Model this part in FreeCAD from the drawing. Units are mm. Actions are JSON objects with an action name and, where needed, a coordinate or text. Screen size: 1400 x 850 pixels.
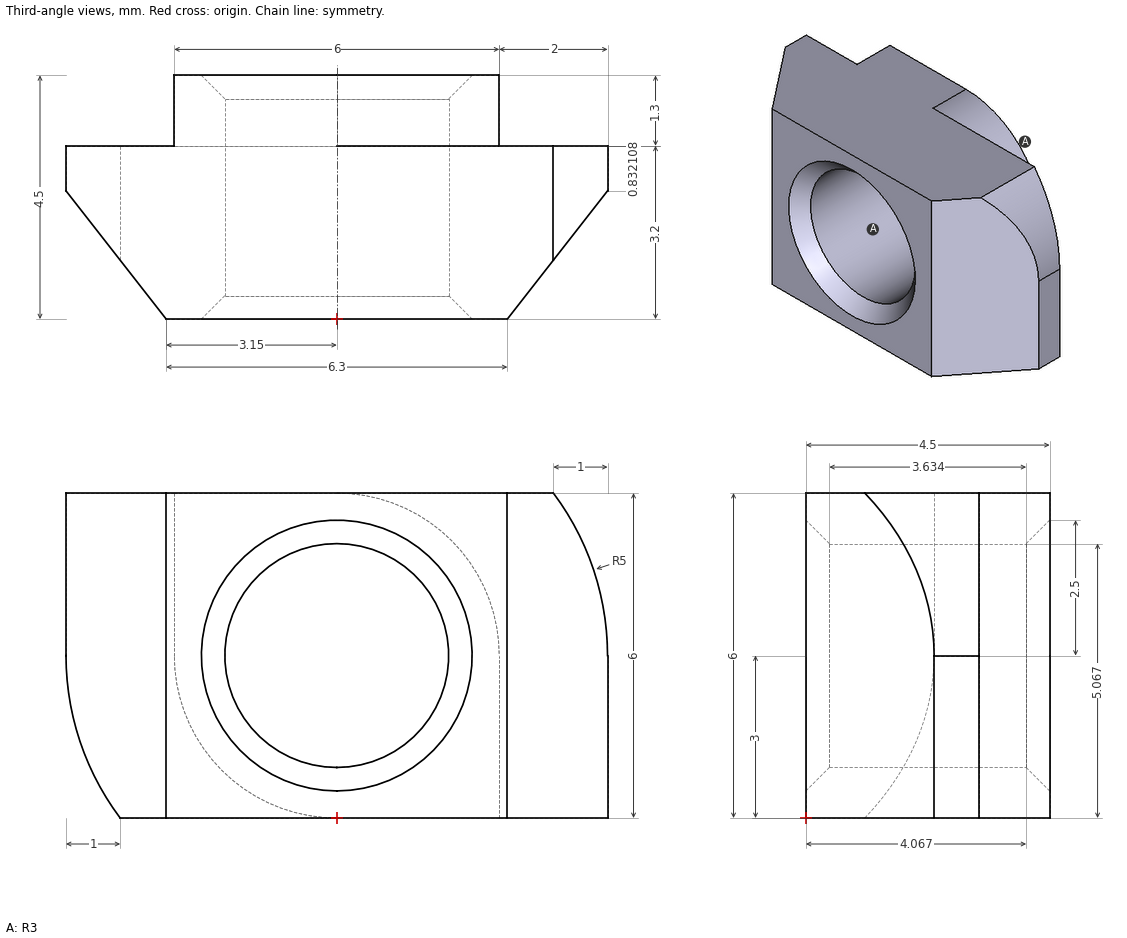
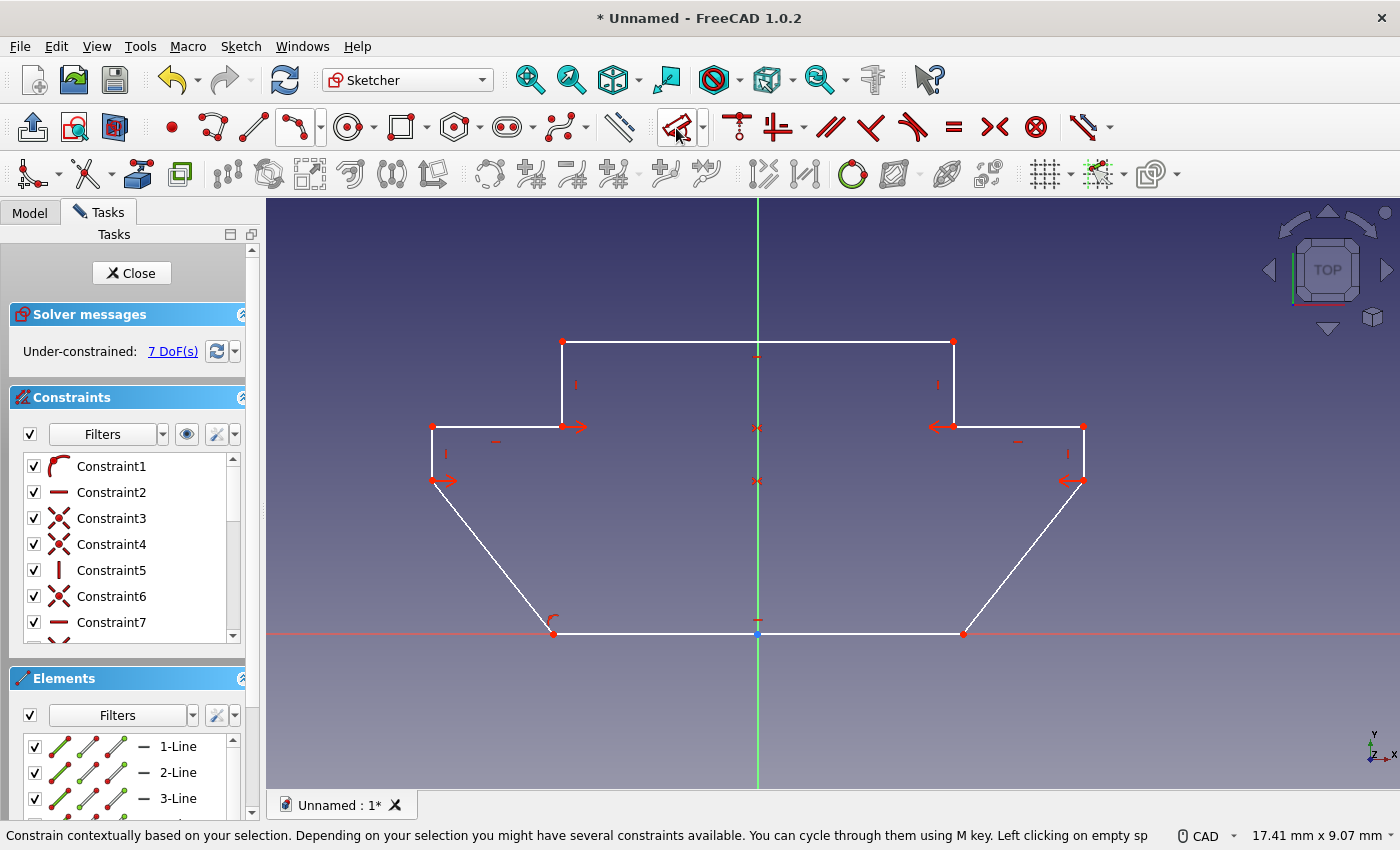
{"action": "left_click", "coordinate": [1045, 427]}
{"action": "left_click", "coordinate": [1019, 393]}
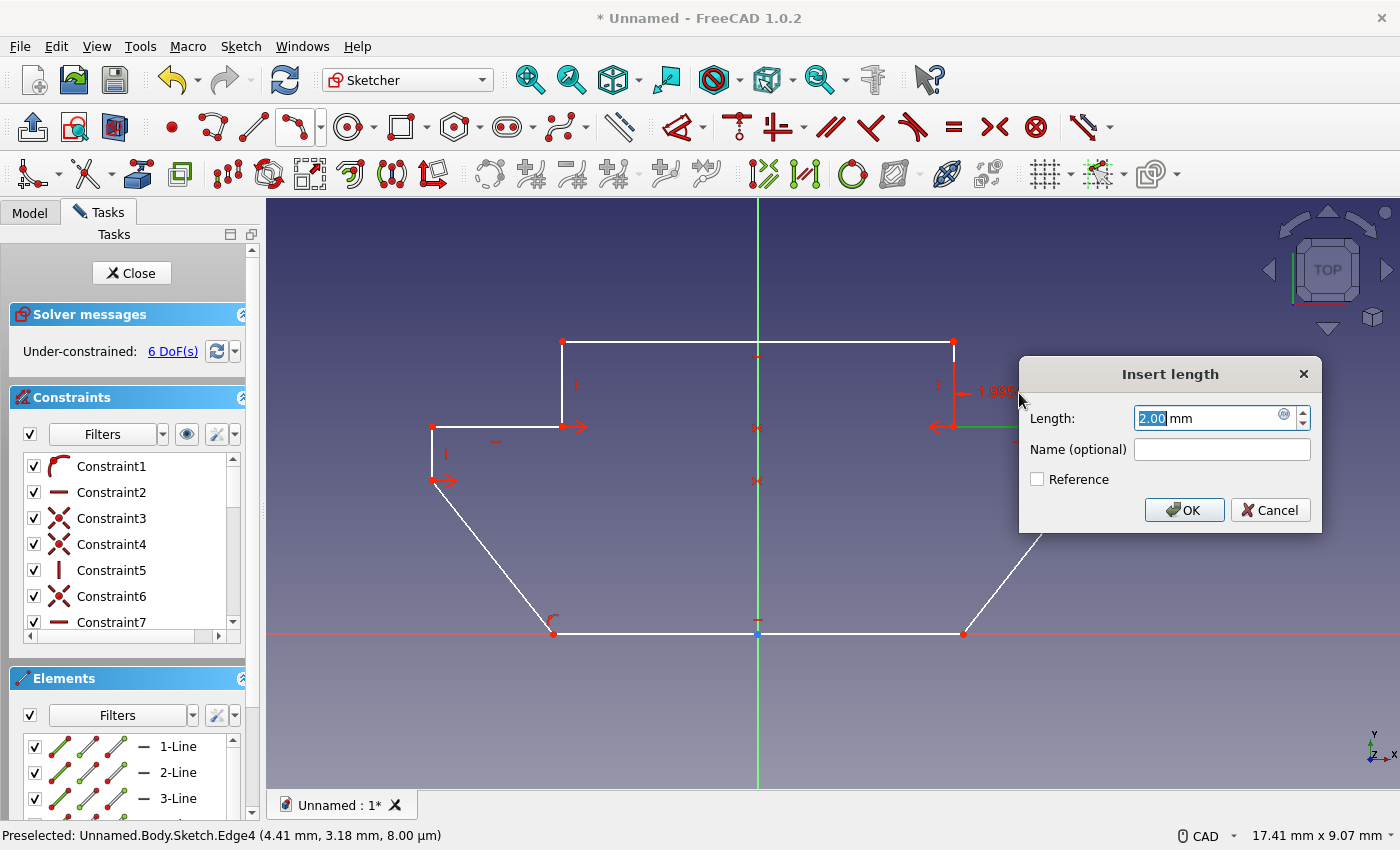
{"action": "type", "text": "2"}
{"action": "key", "text": "Return"}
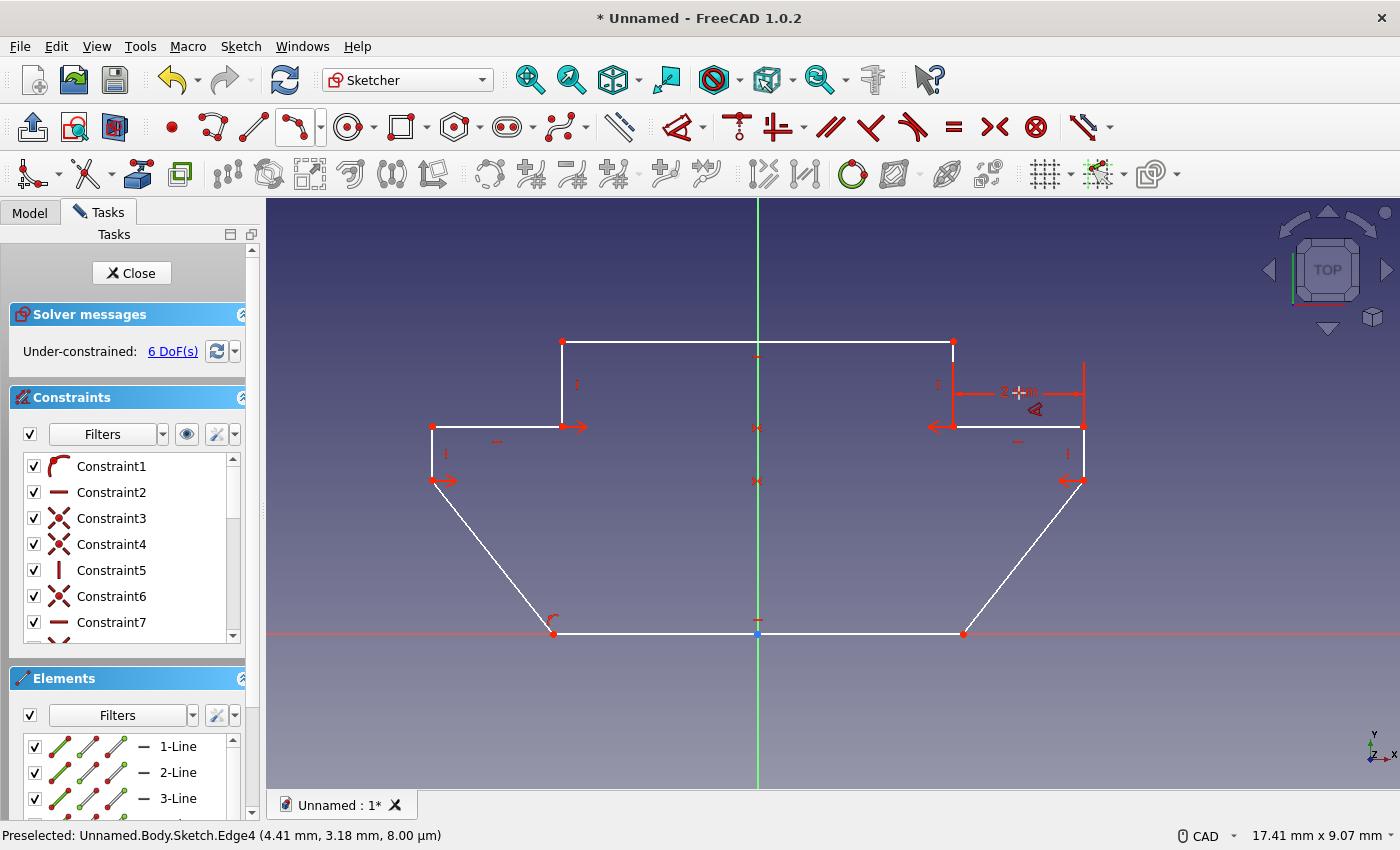
{"action": "left_click", "coordinate": [836, 342]}
{"action": "left_click", "coordinate": [668, 308]}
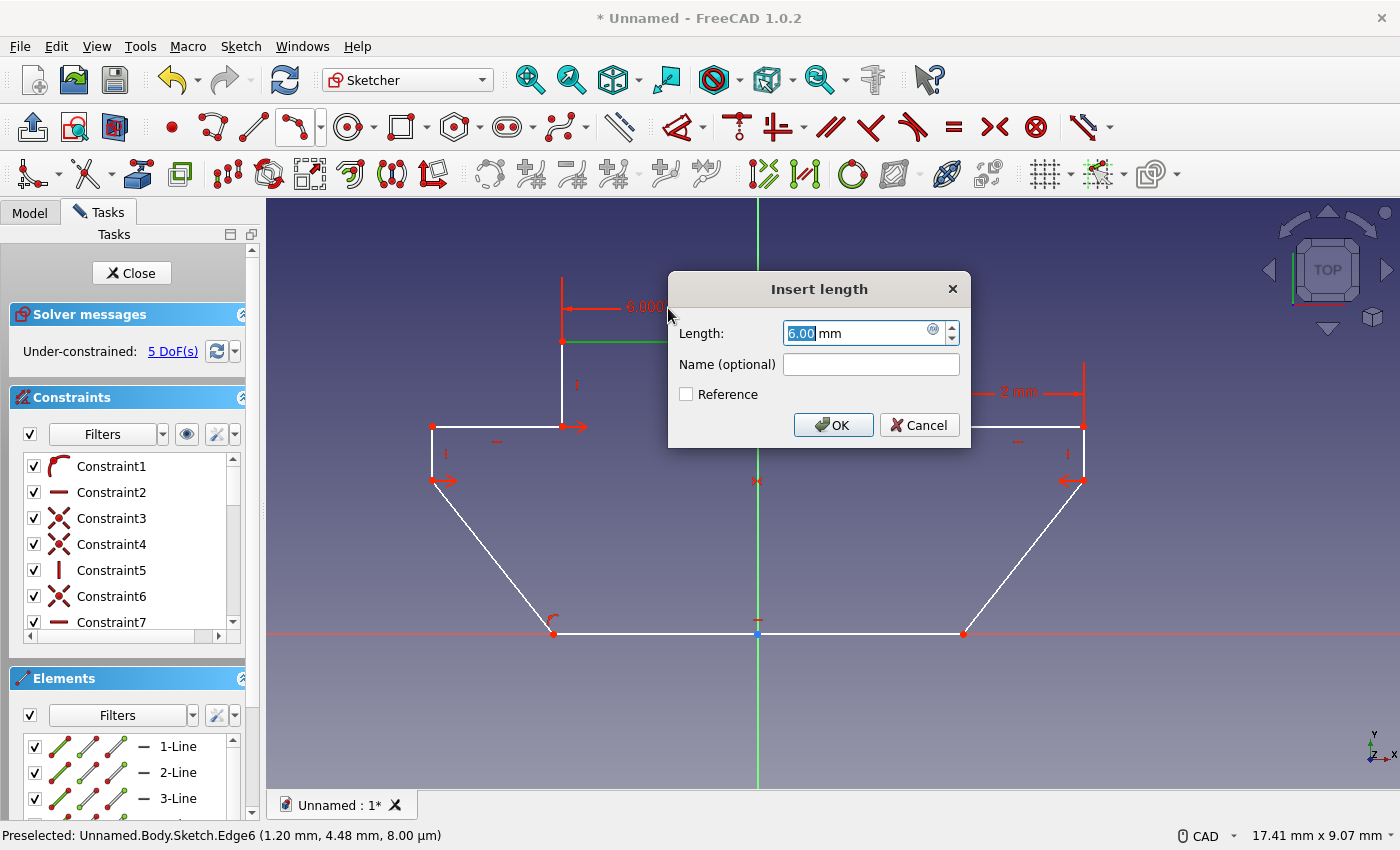
{"action": "type", "text": "6"}
{"action": "key", "text": "Return"}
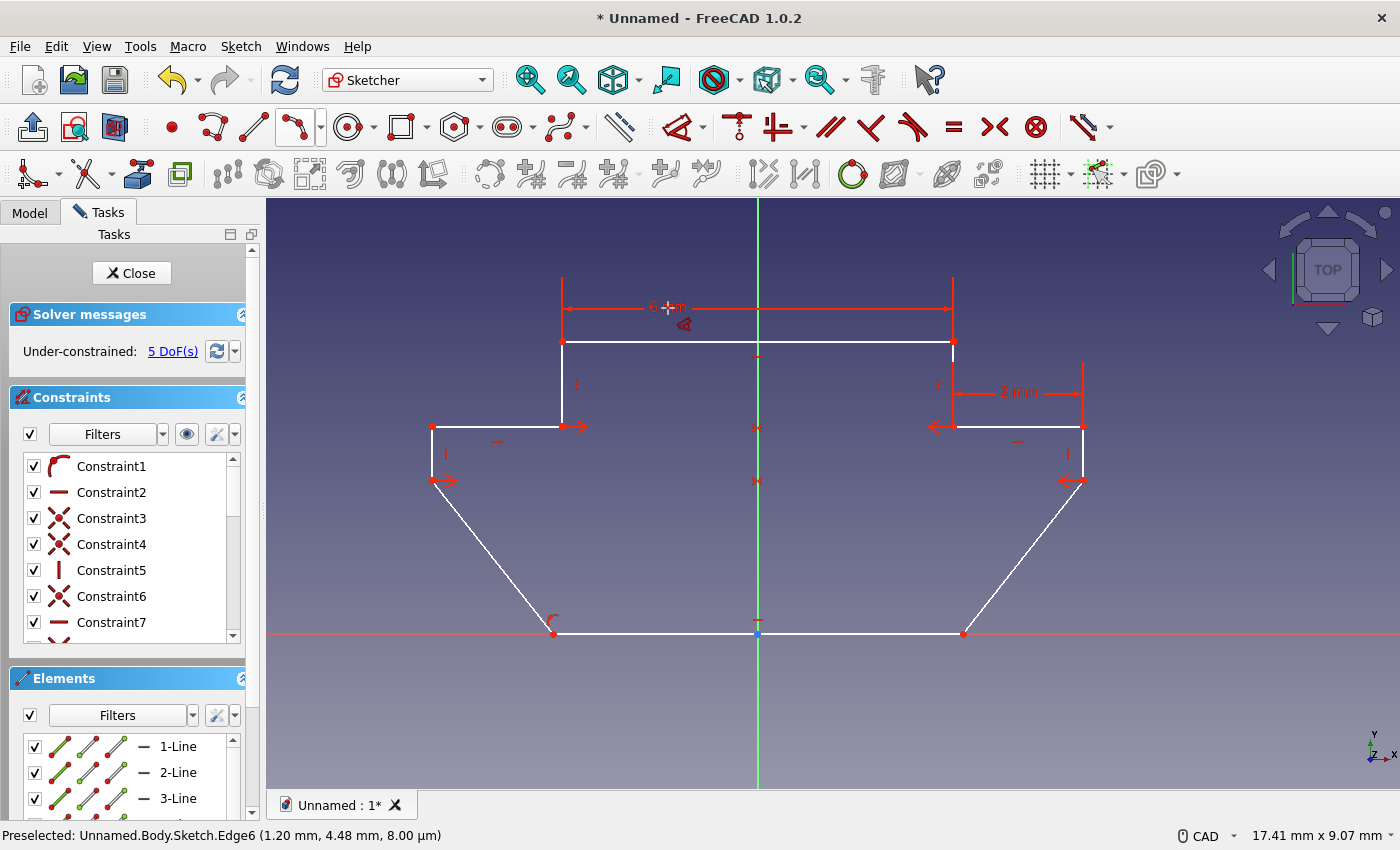
{"action": "left_click", "coordinate": [676, 634]}
{"action": "left_click", "coordinate": [664, 668]}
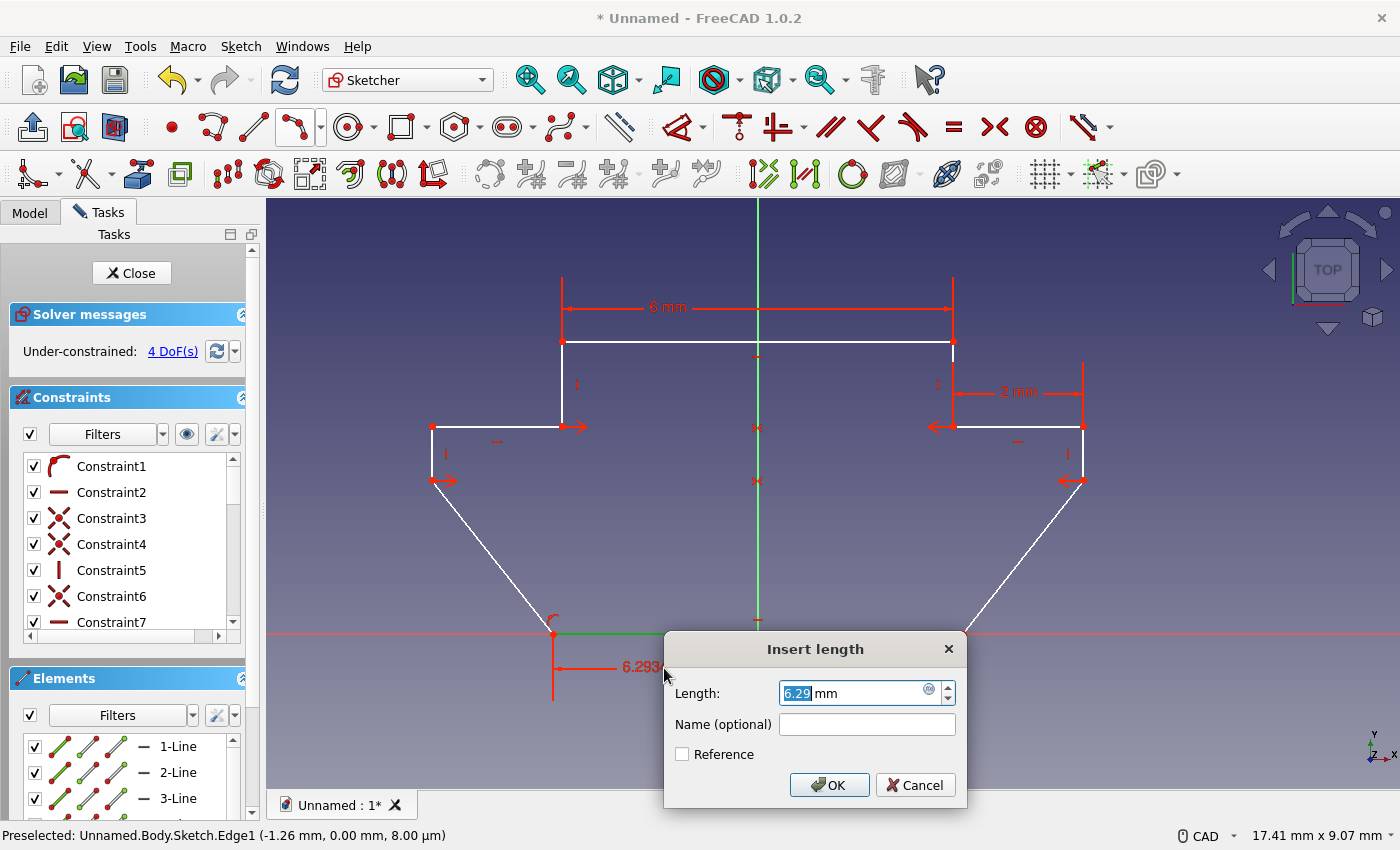
{"action": "type", "text": "6.3"}
{"action": "key", "text": "Return"}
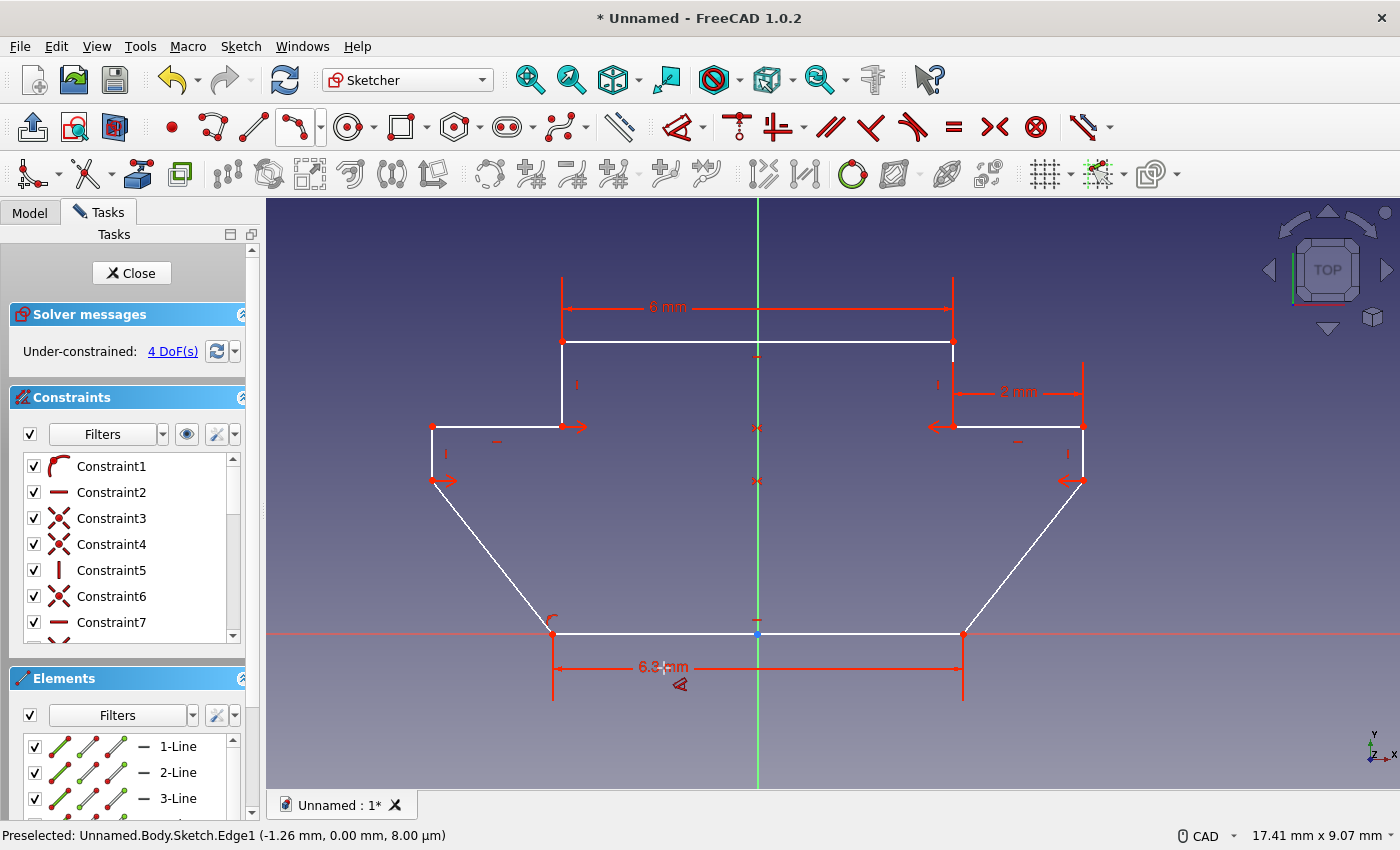
{"action": "left_click", "coordinate": [953, 402]}
{"action": "left_click", "coordinate": [987, 365]}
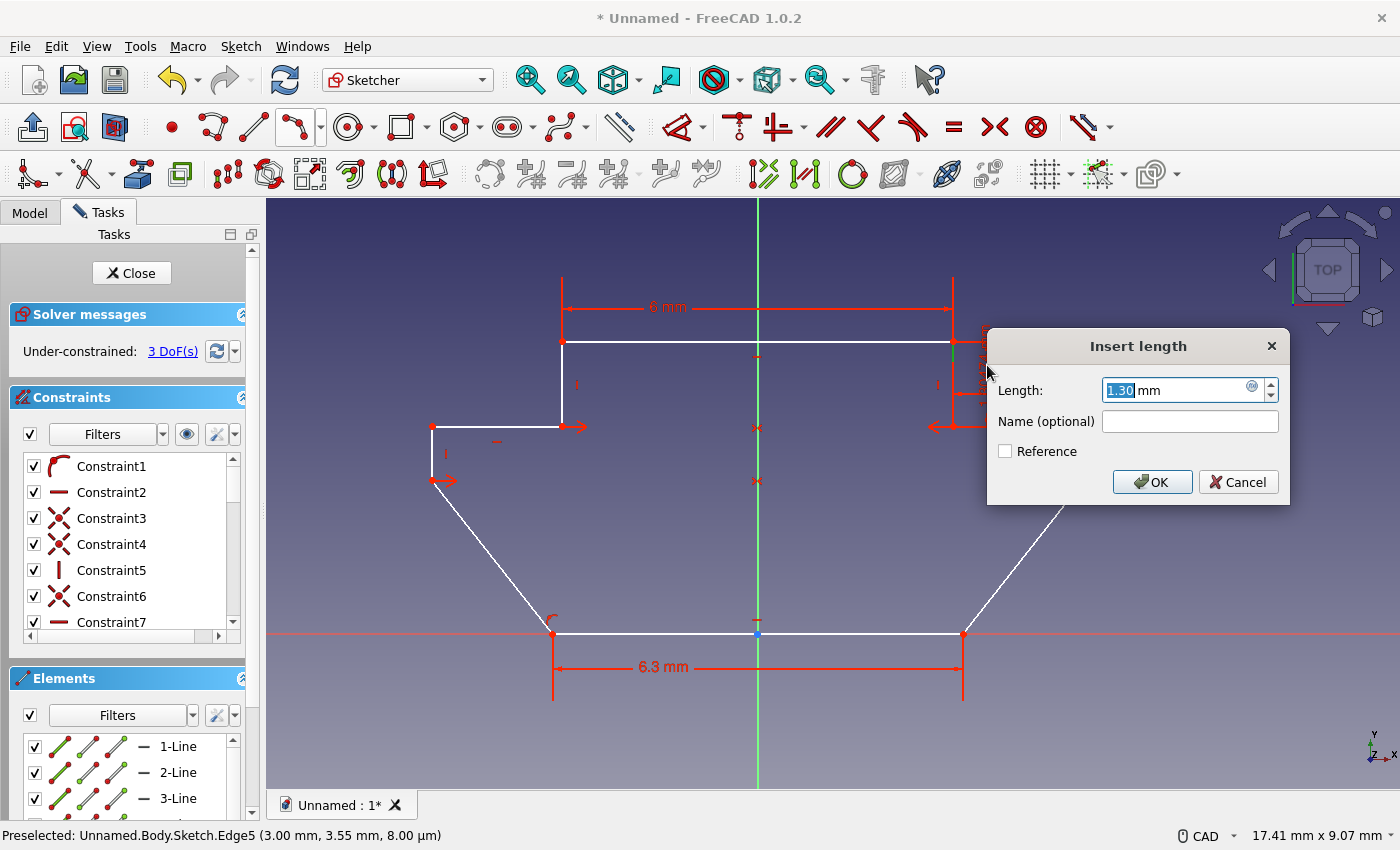
{"action": "type", "text": "1.3"}
{"action": "key", "text": "Return"}